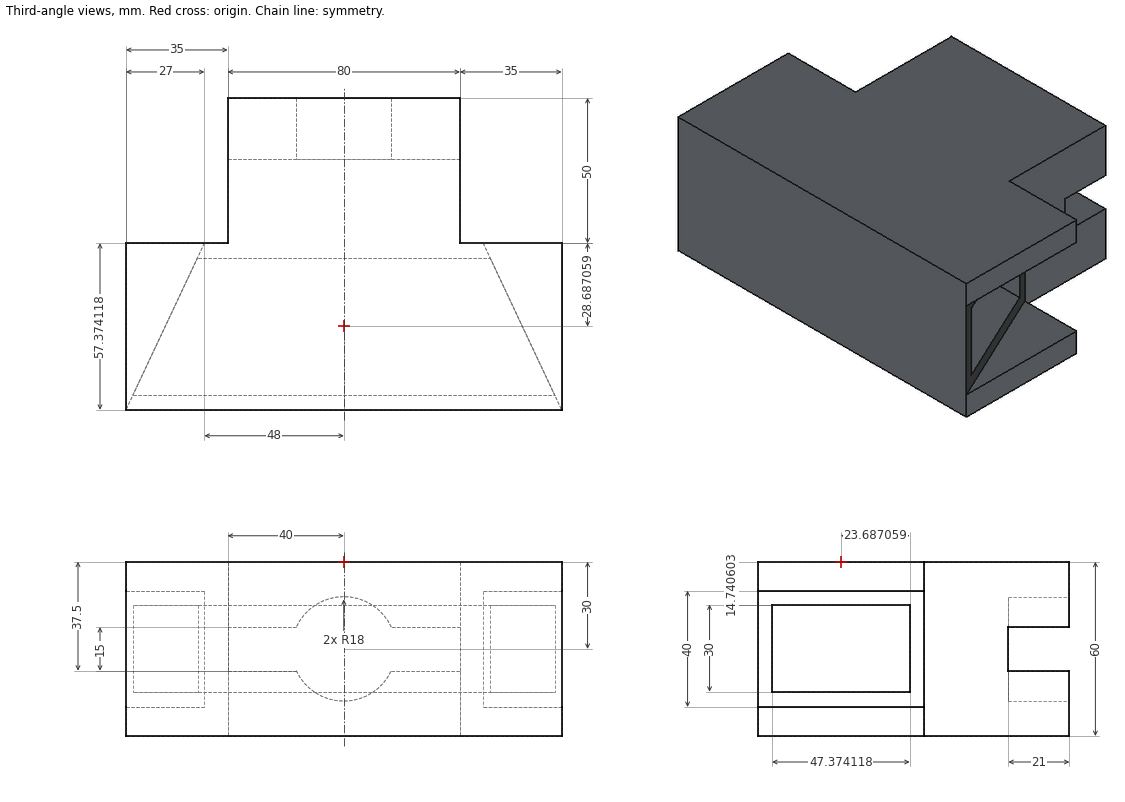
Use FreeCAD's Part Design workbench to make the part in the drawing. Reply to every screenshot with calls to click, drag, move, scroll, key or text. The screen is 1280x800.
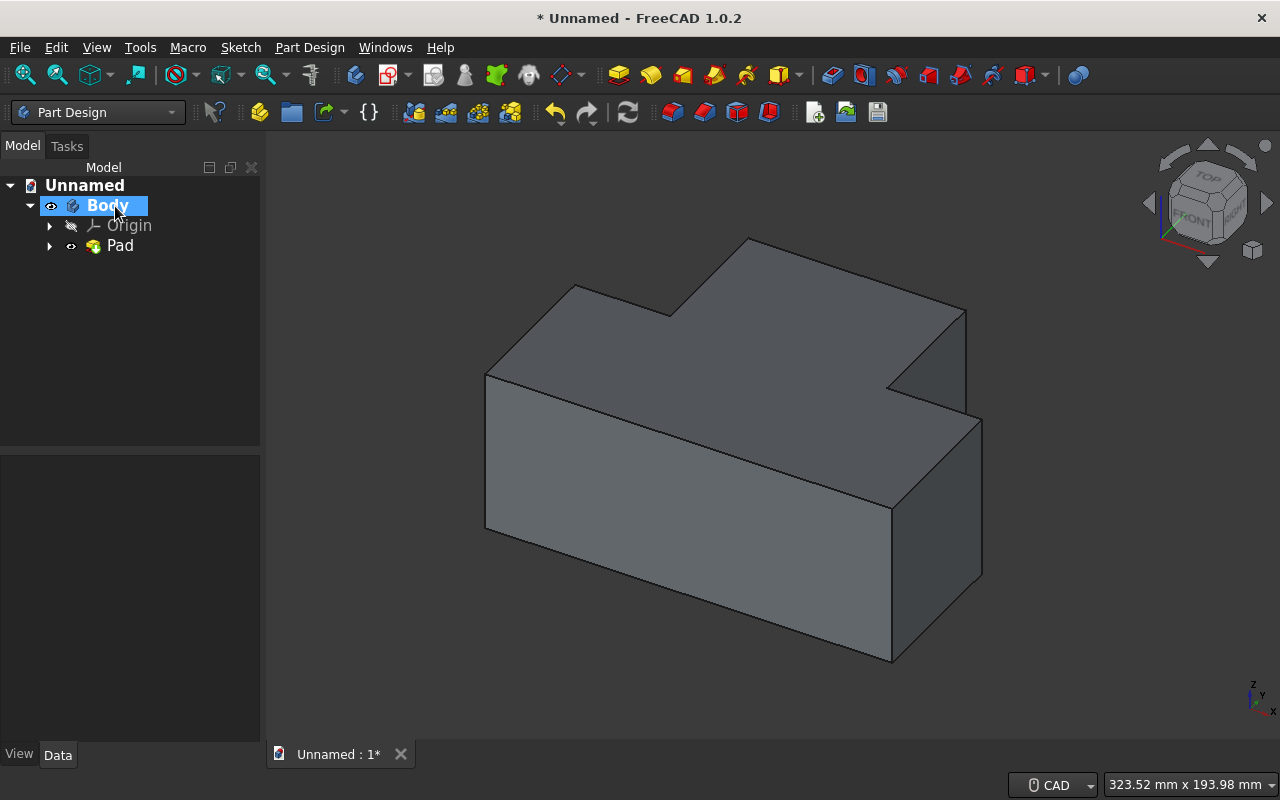
key(4)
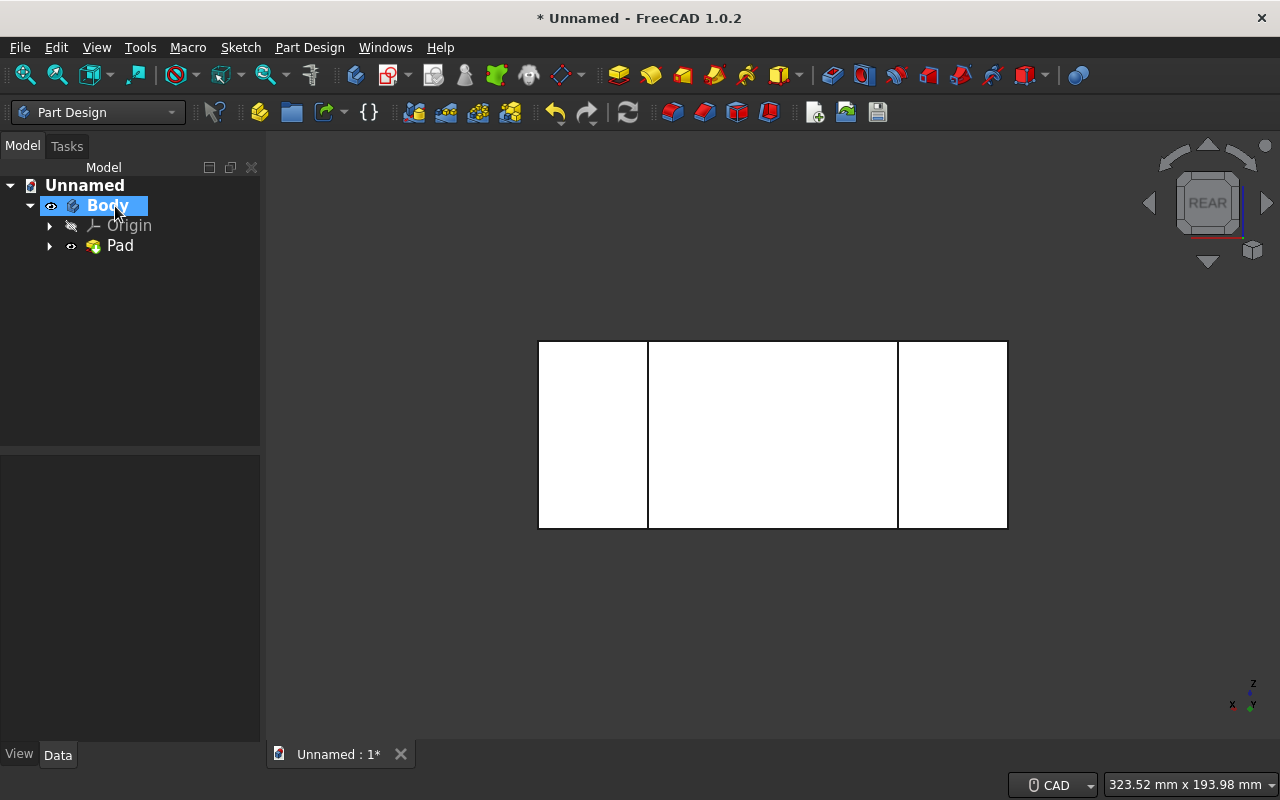
click(773, 434)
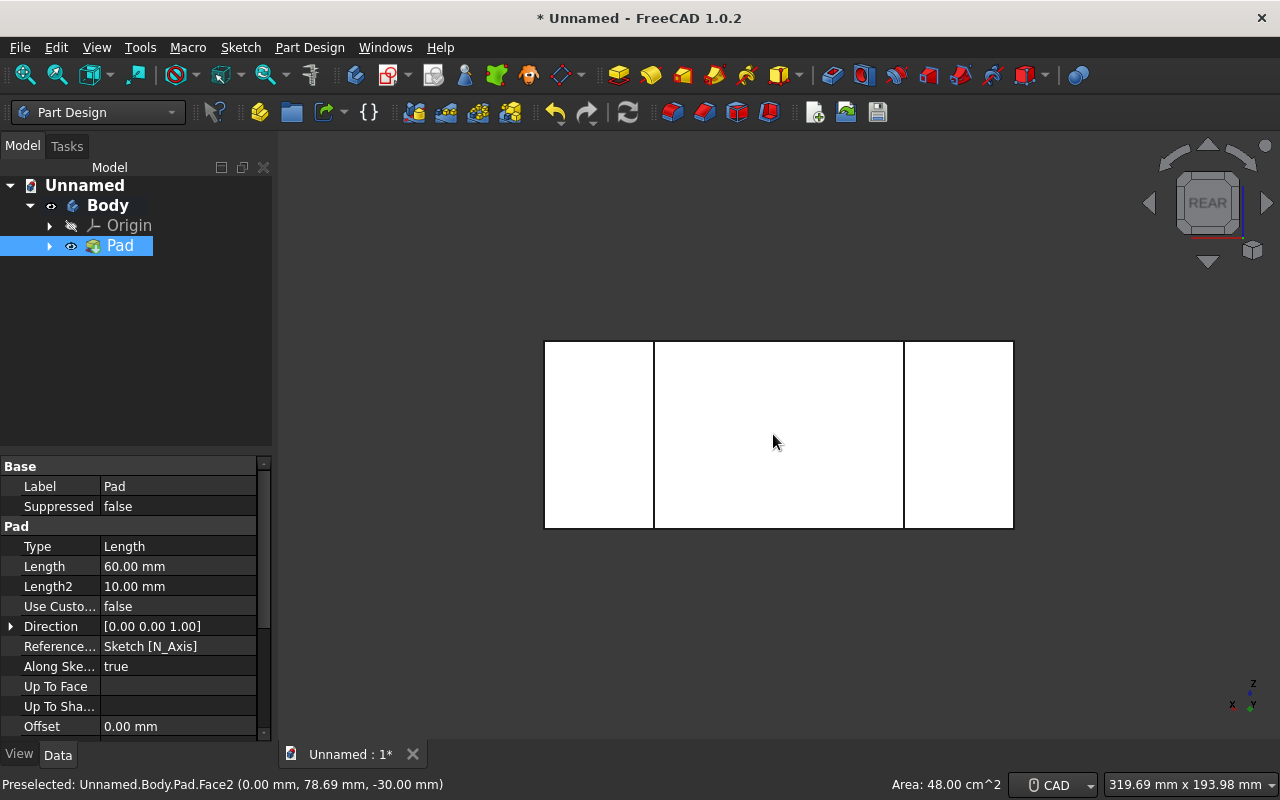
click(388, 76)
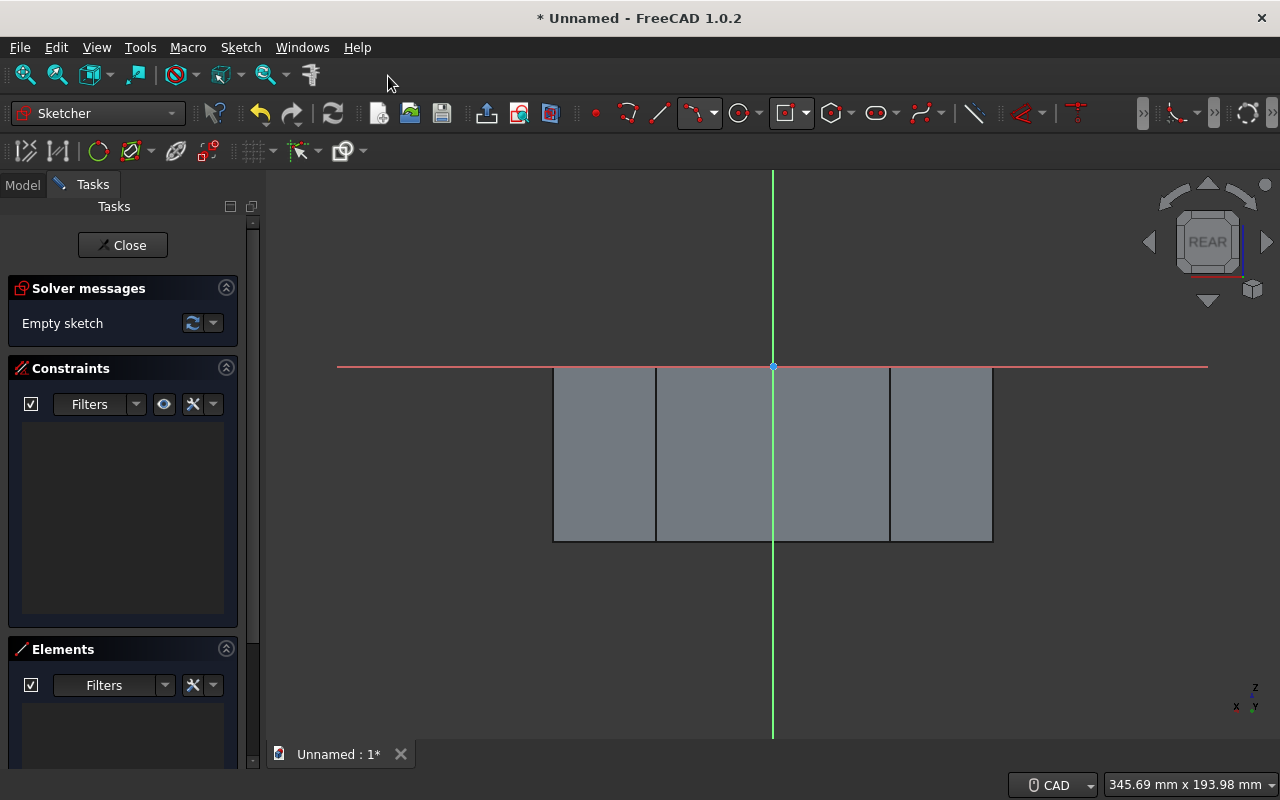
scroll(813, 427, up, 5)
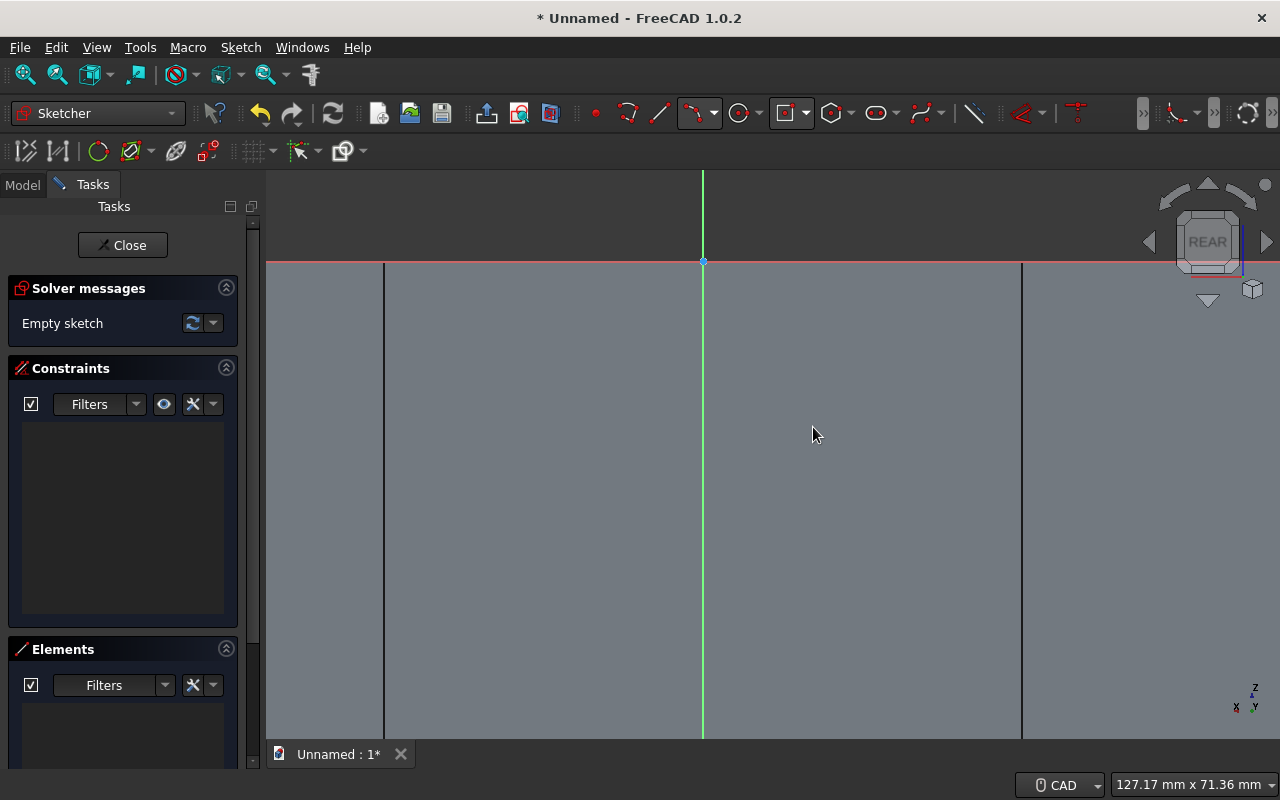
key(g)
key(m)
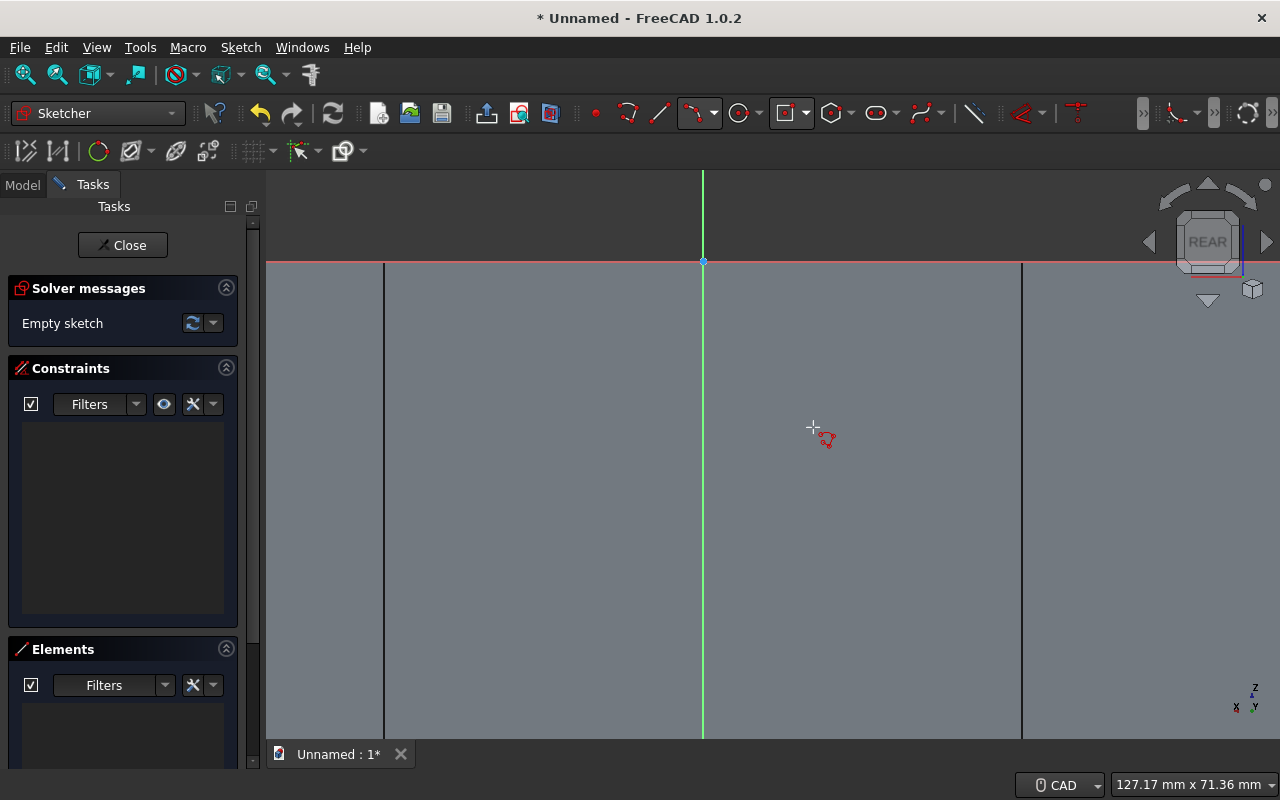
click(834, 561)
click(1022, 561)
click(1022, 441)
click(834, 441)
right_click(834, 441)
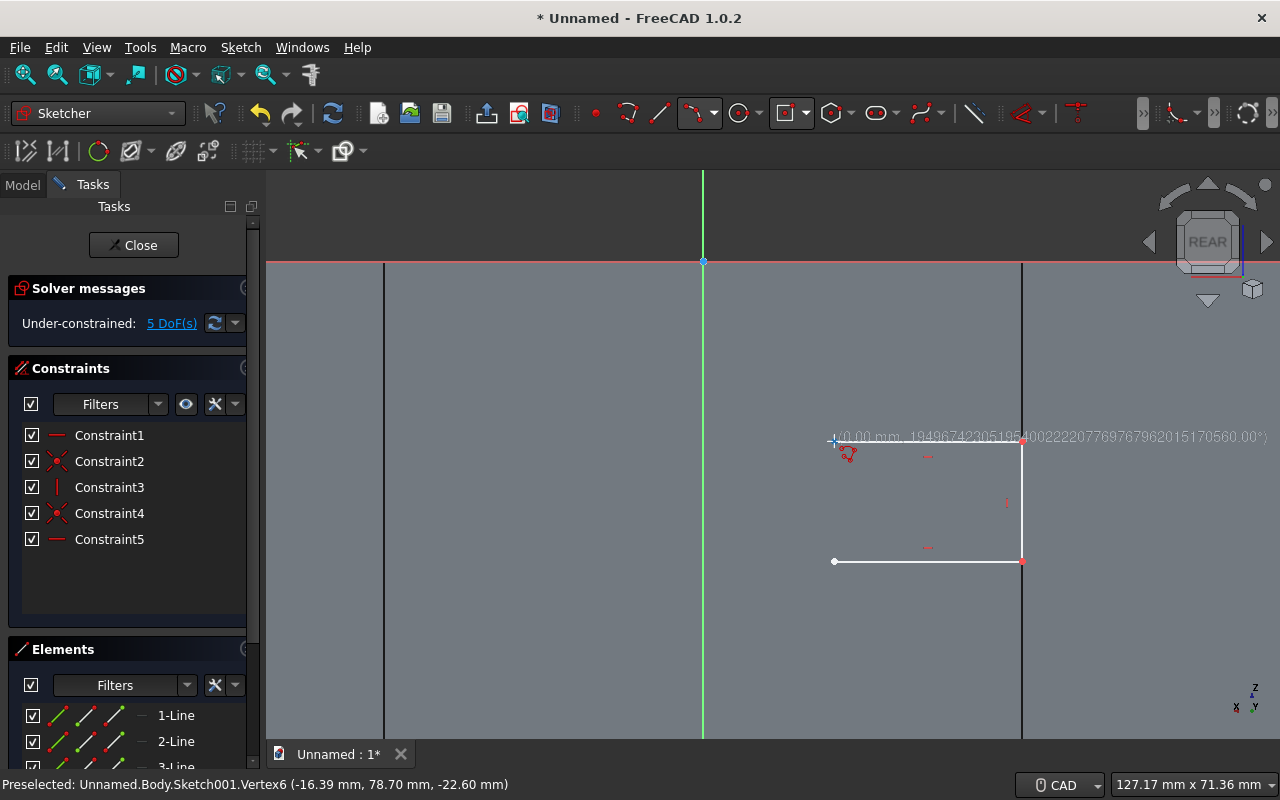
click(573, 441)
click(384, 441)
click(384, 561)
click(573, 561)
right_click(573, 561)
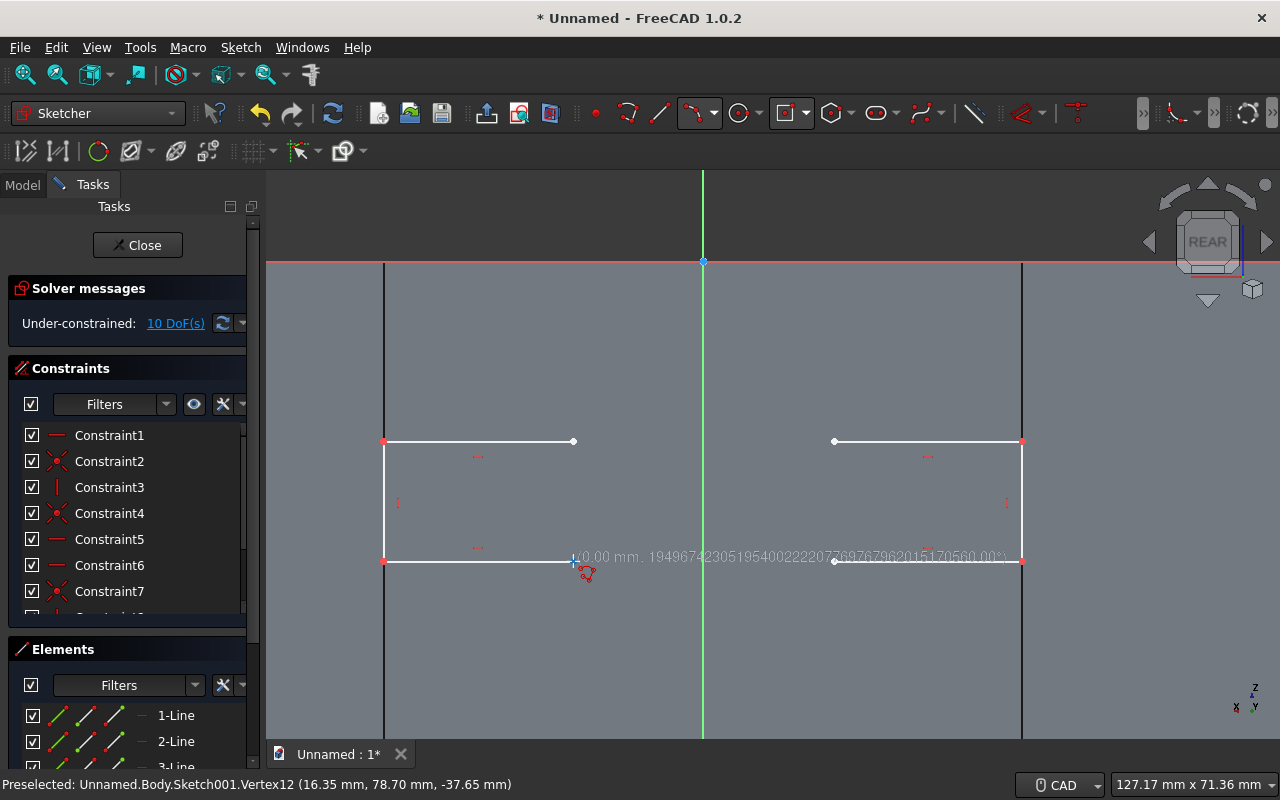
key(g)
key(3)
key(a)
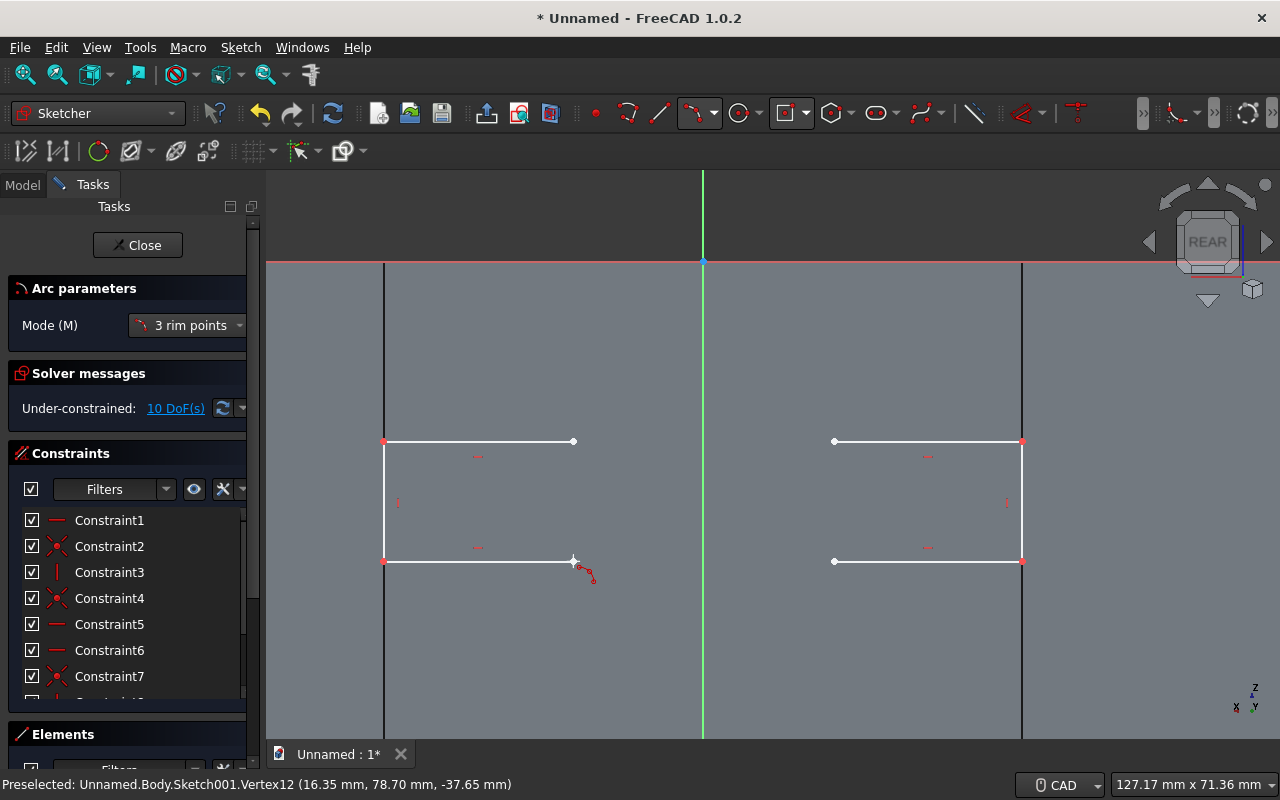
click(834, 442)
click(573, 442)
click(736, 361)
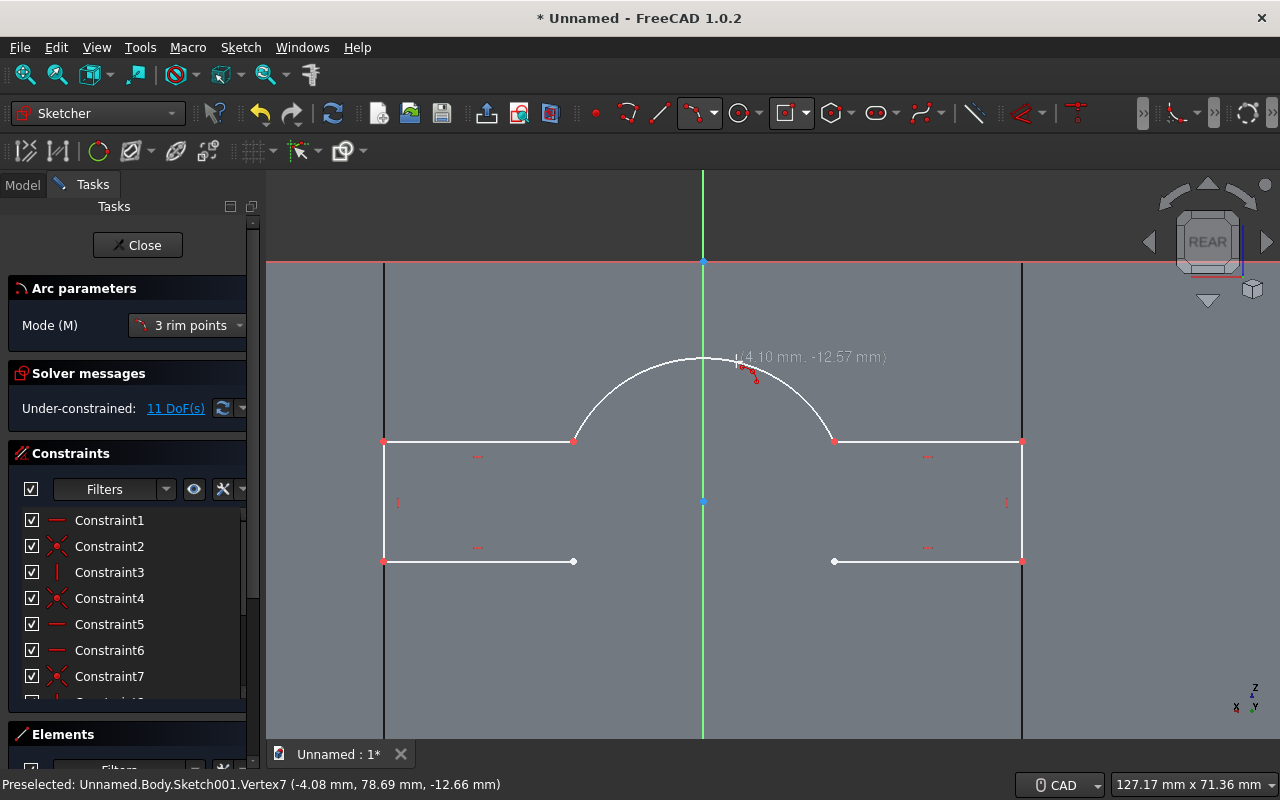
click(573, 562)
click(834, 562)
click(671, 641)
key(Escape)